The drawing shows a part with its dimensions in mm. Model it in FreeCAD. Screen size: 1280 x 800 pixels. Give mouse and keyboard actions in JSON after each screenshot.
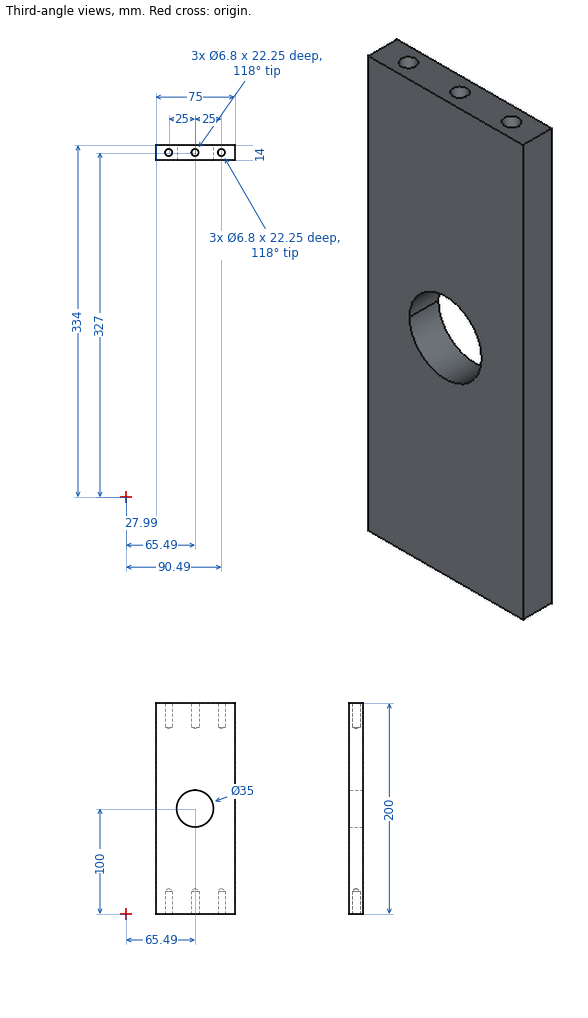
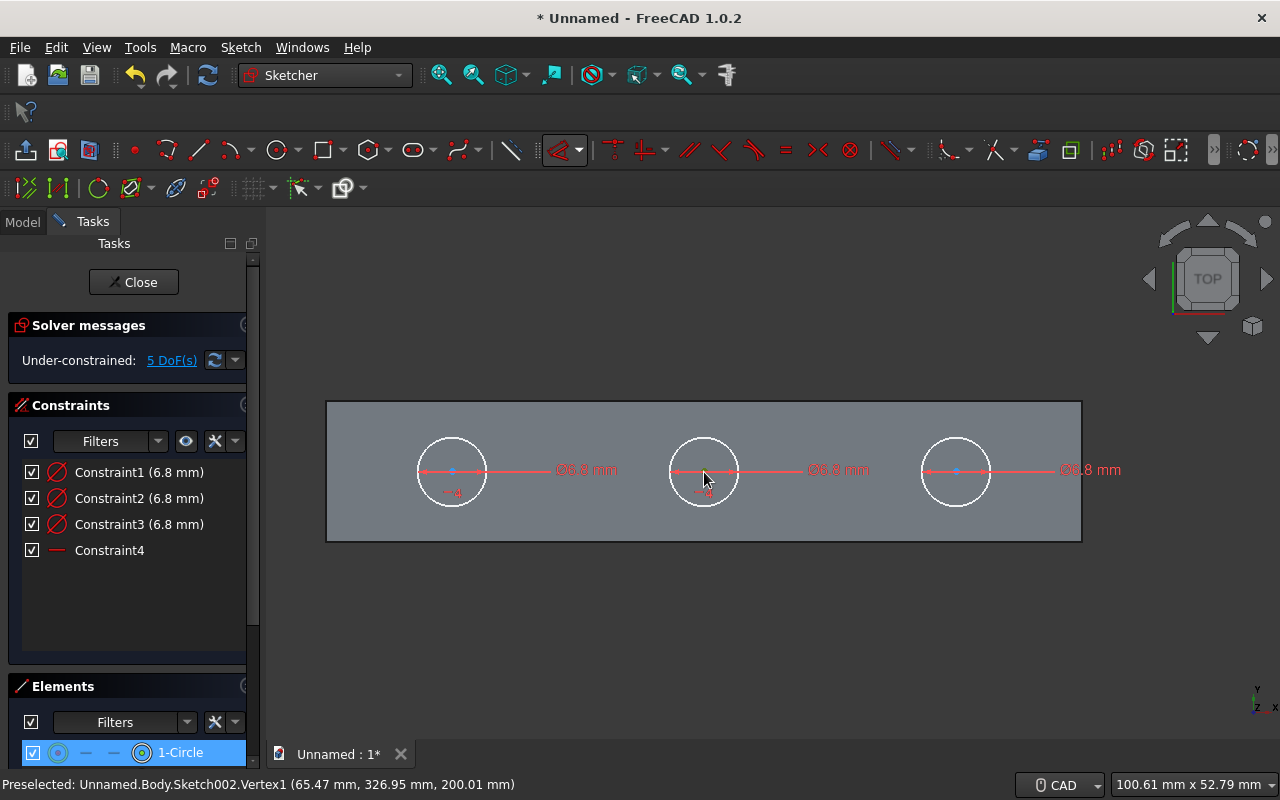
{"action": "left_click", "coordinate": [956, 472]}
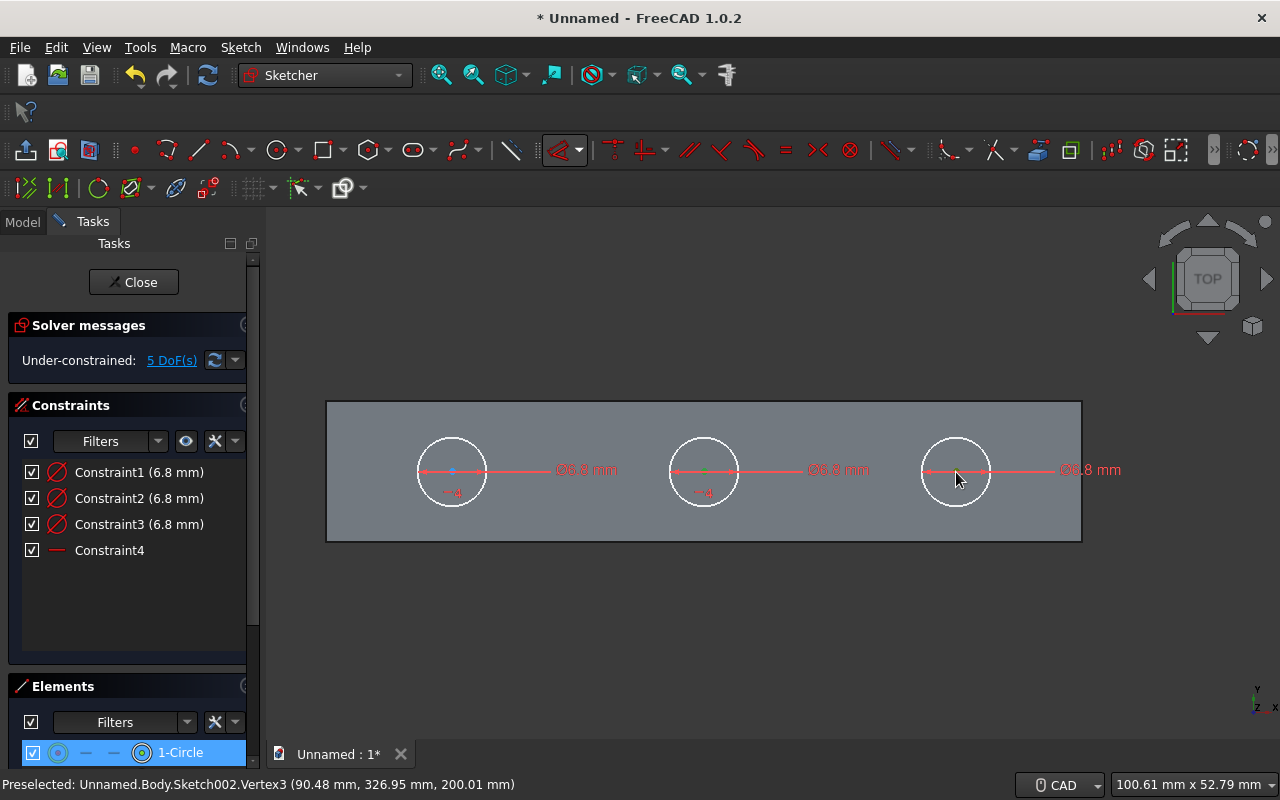
{"action": "left_click", "coordinate": [668, 150]}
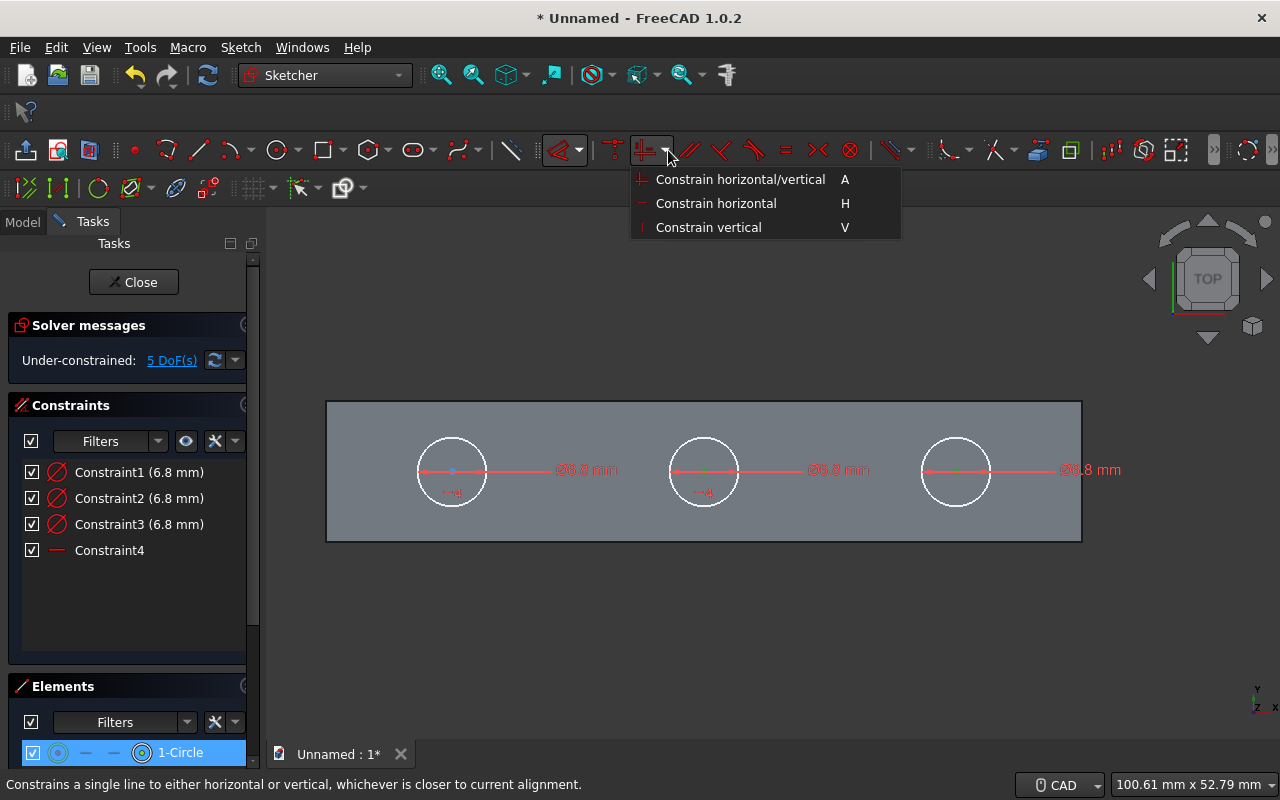
{"action": "left_click", "coordinate": [766, 203]}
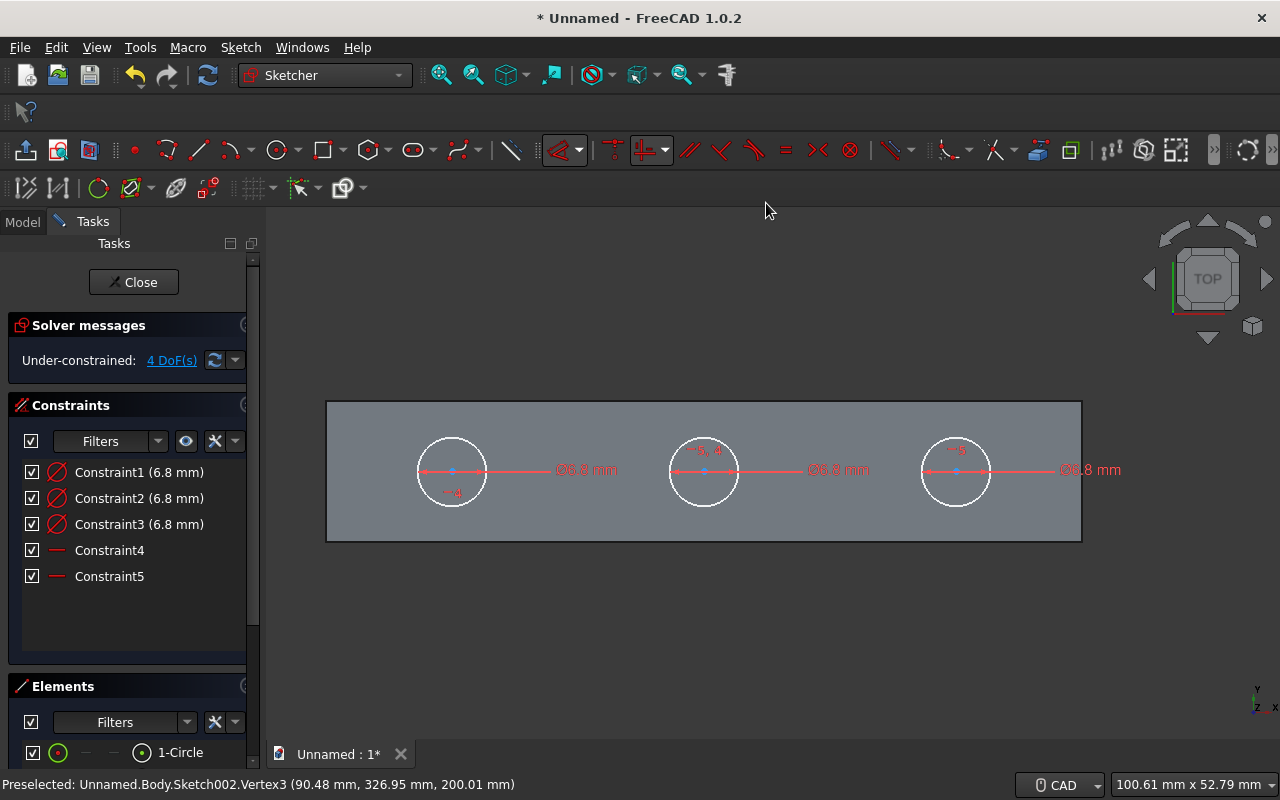
{"action": "left_click", "coordinate": [704, 472]}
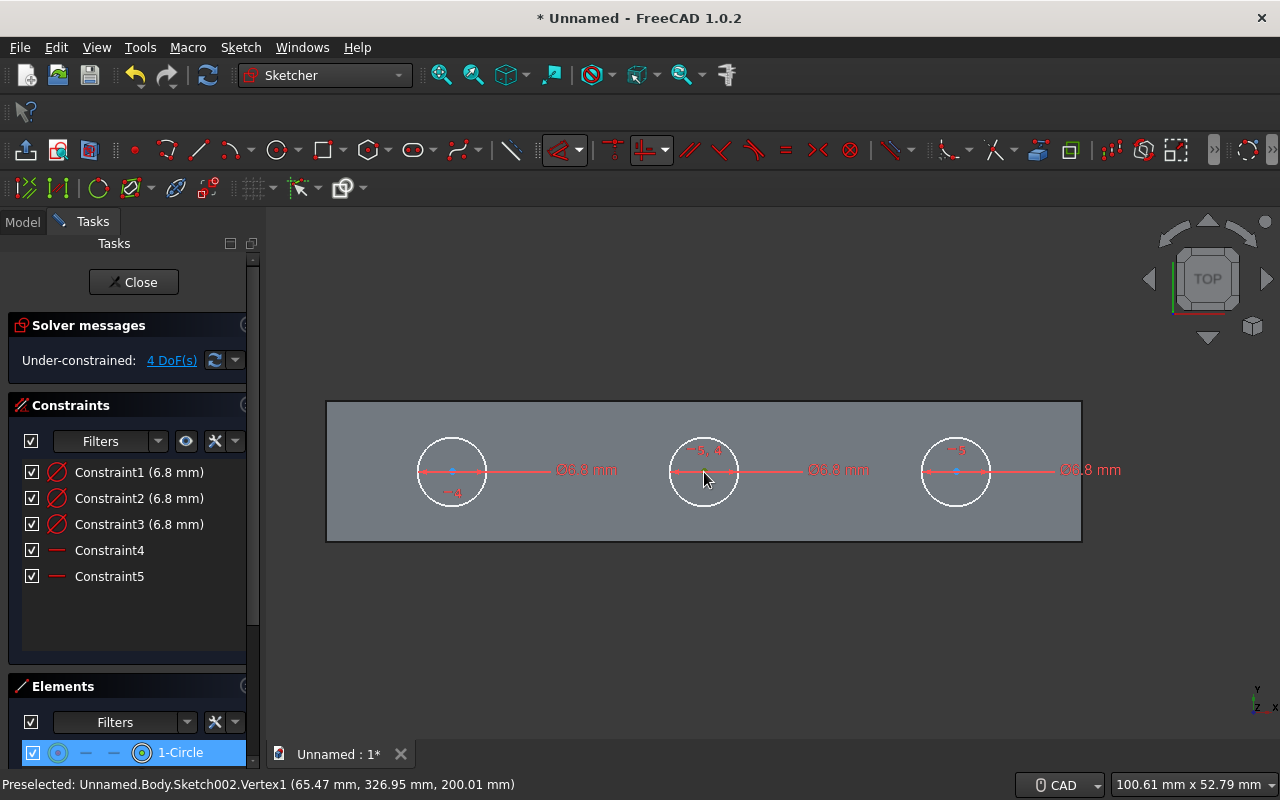
{"action": "left_click", "coordinate": [582, 150]}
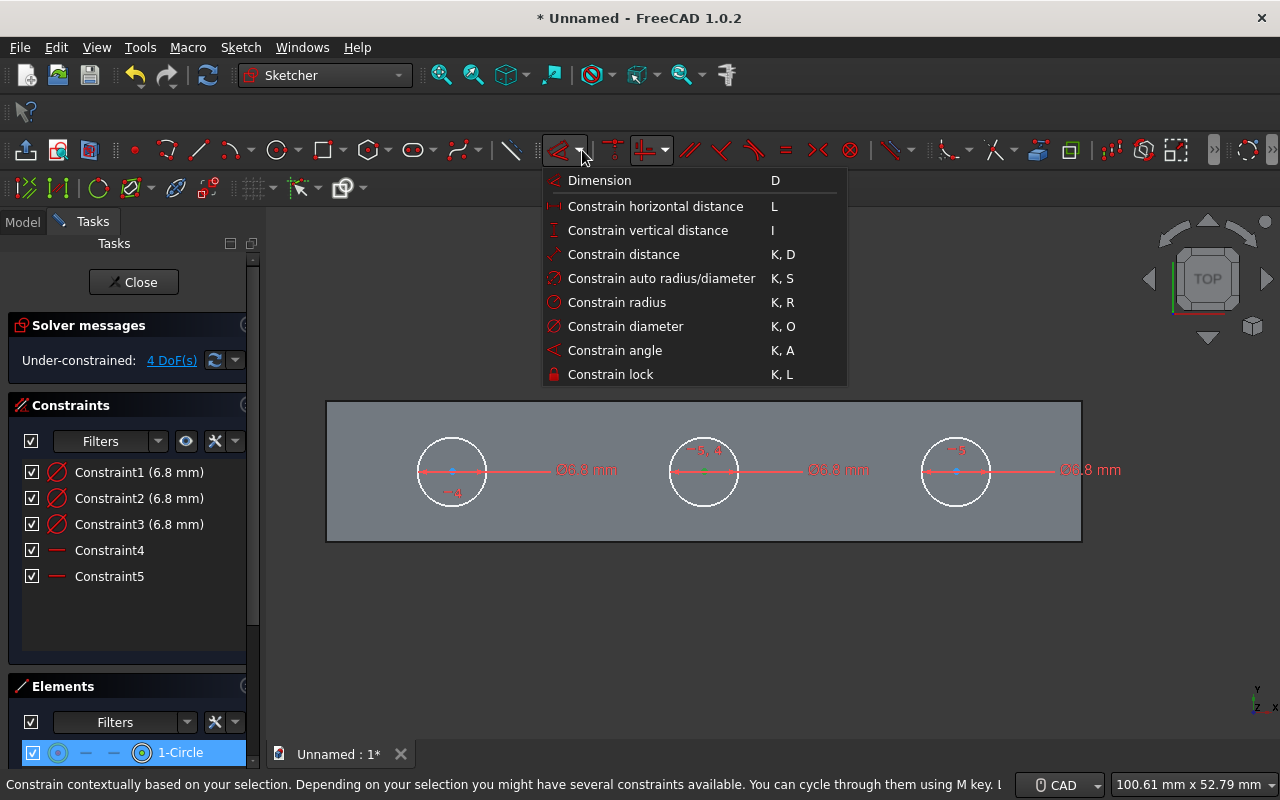
{"action": "left_click", "coordinate": [695, 230]}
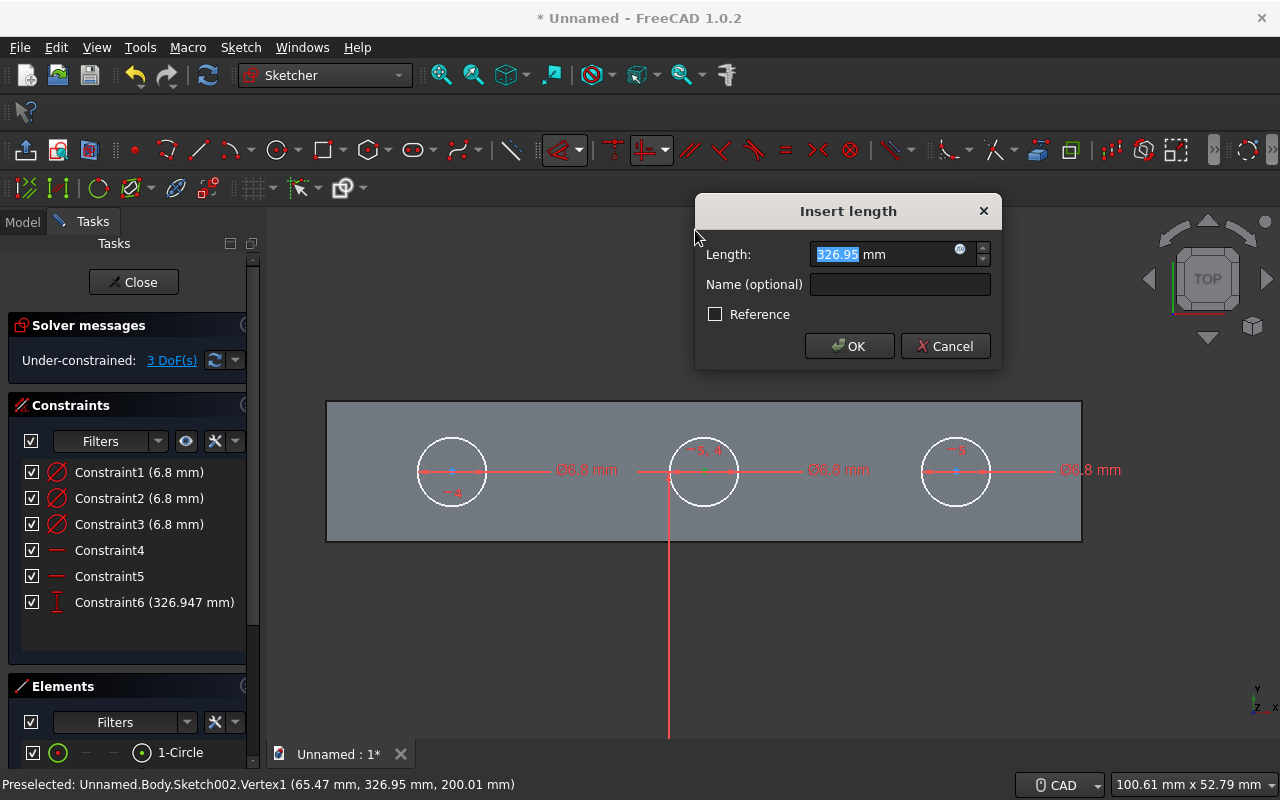
{"action": "type", "text": "327"}
{"action": "key", "text": "Return"}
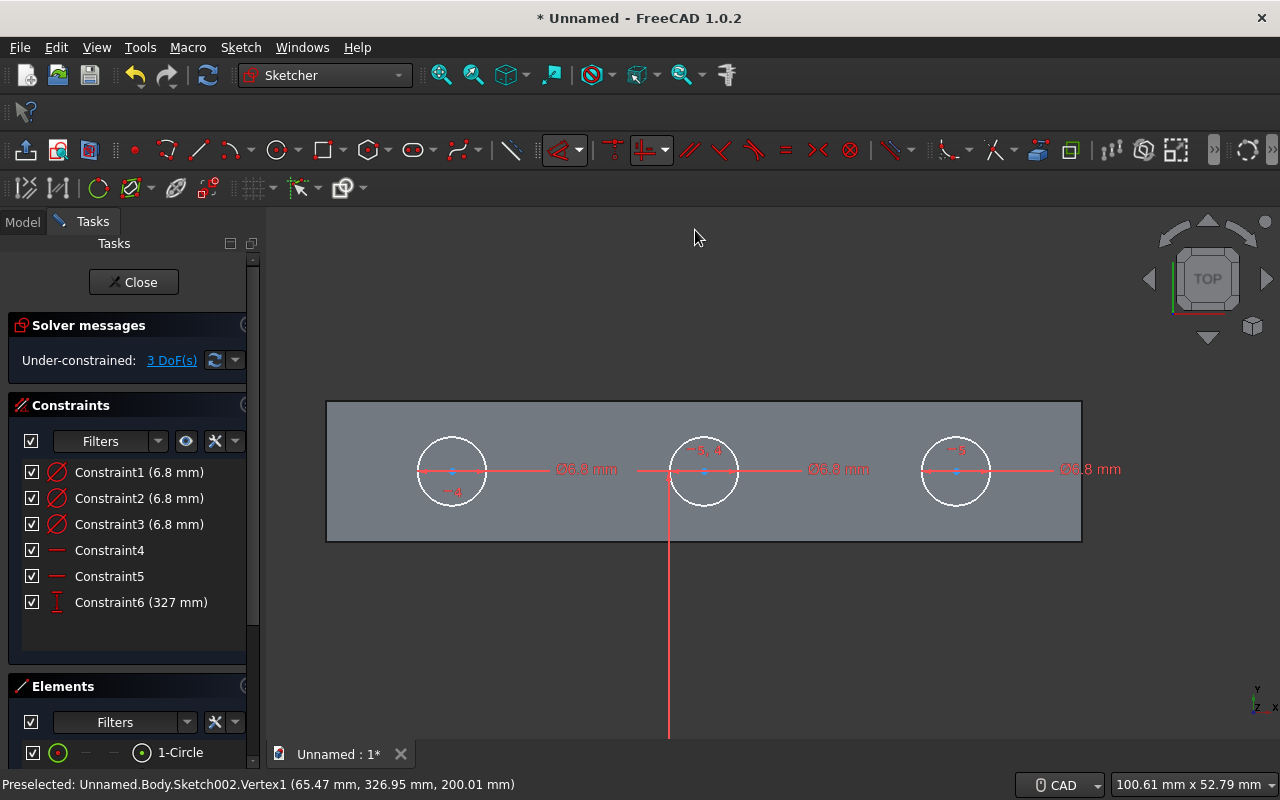
{"action": "left_click", "coordinate": [704, 471]}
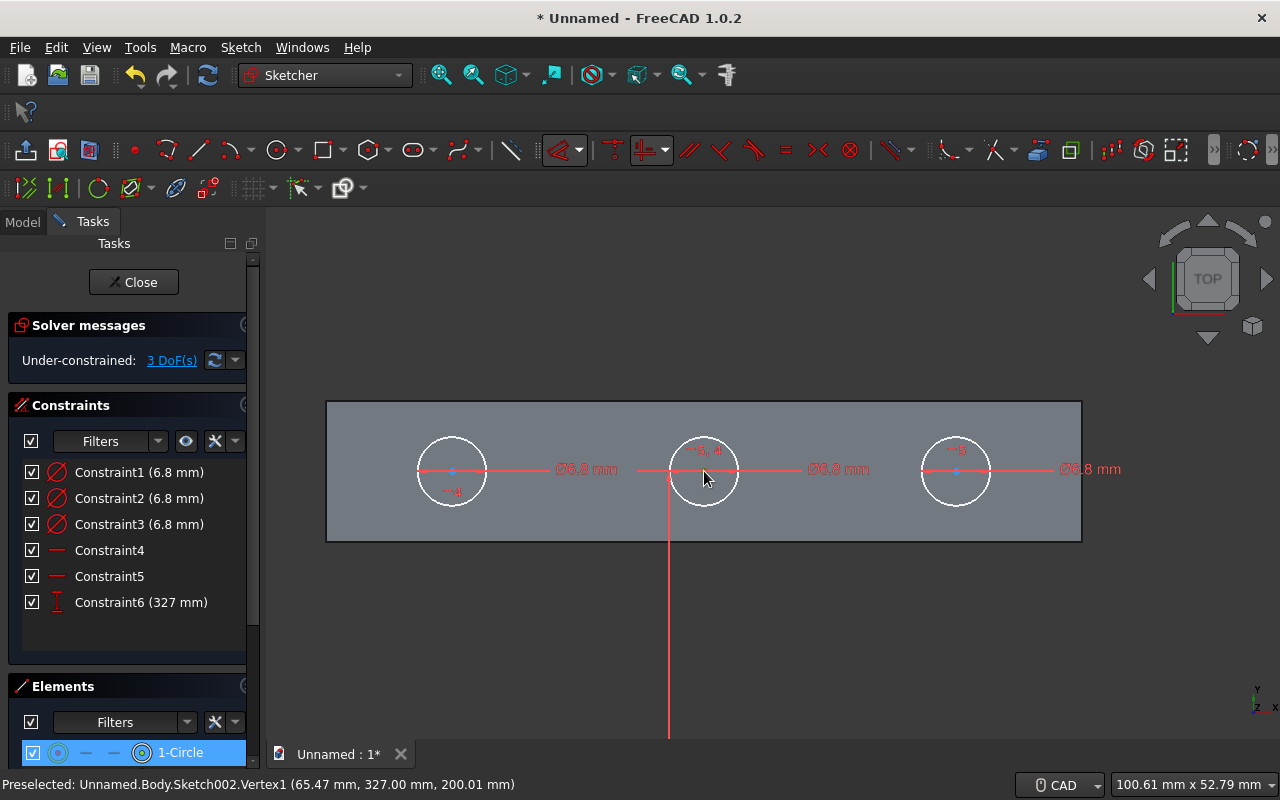
{"action": "left_click", "coordinate": [452, 471]}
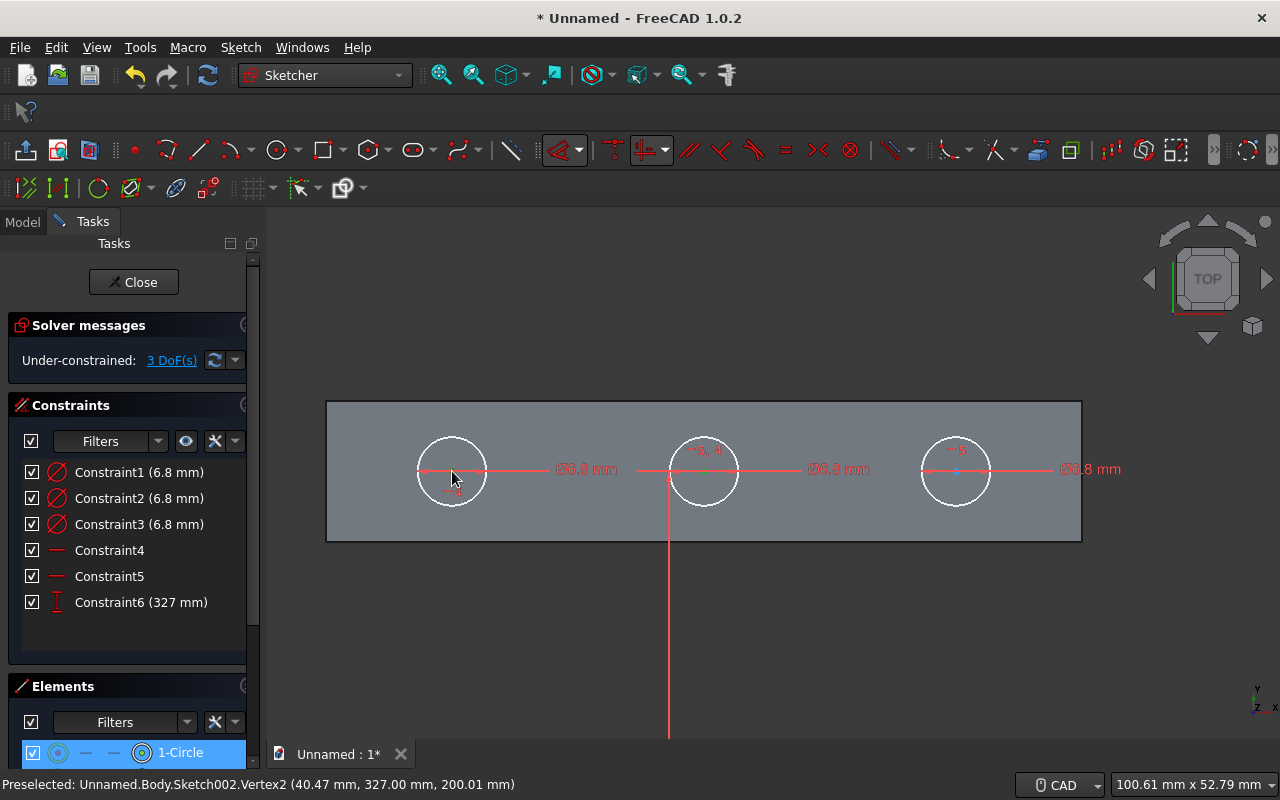
{"action": "key", "text": "l"}